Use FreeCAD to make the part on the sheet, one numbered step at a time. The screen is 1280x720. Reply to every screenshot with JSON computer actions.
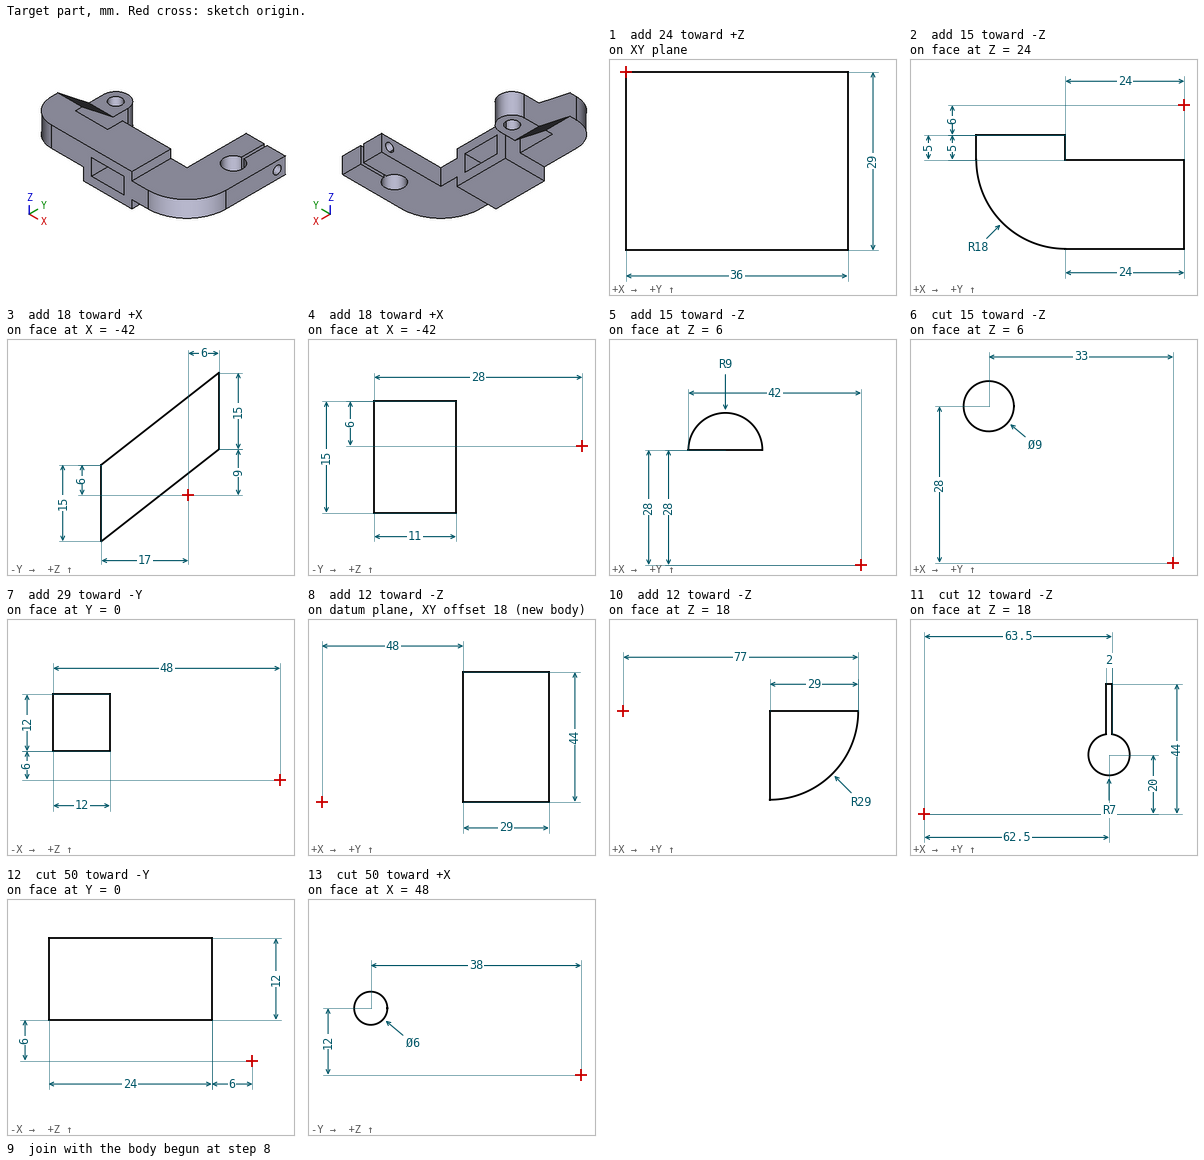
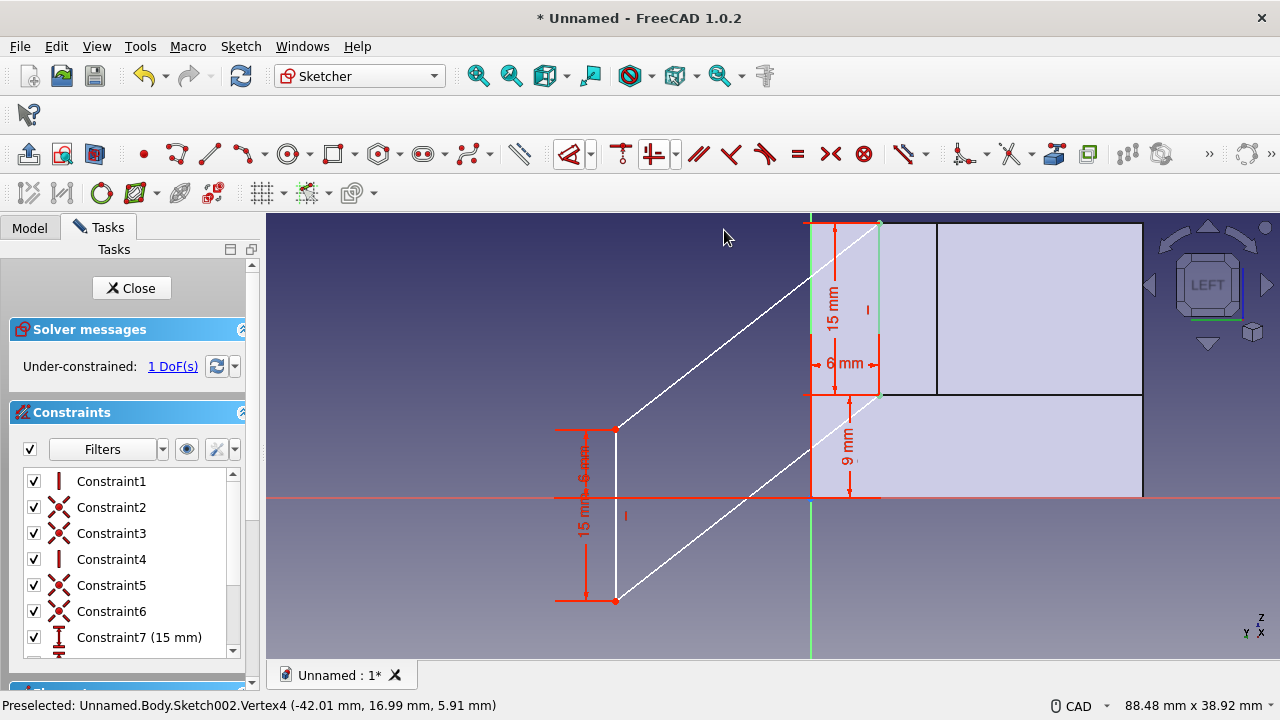
{"action": "left_click", "coordinate": [616, 430]}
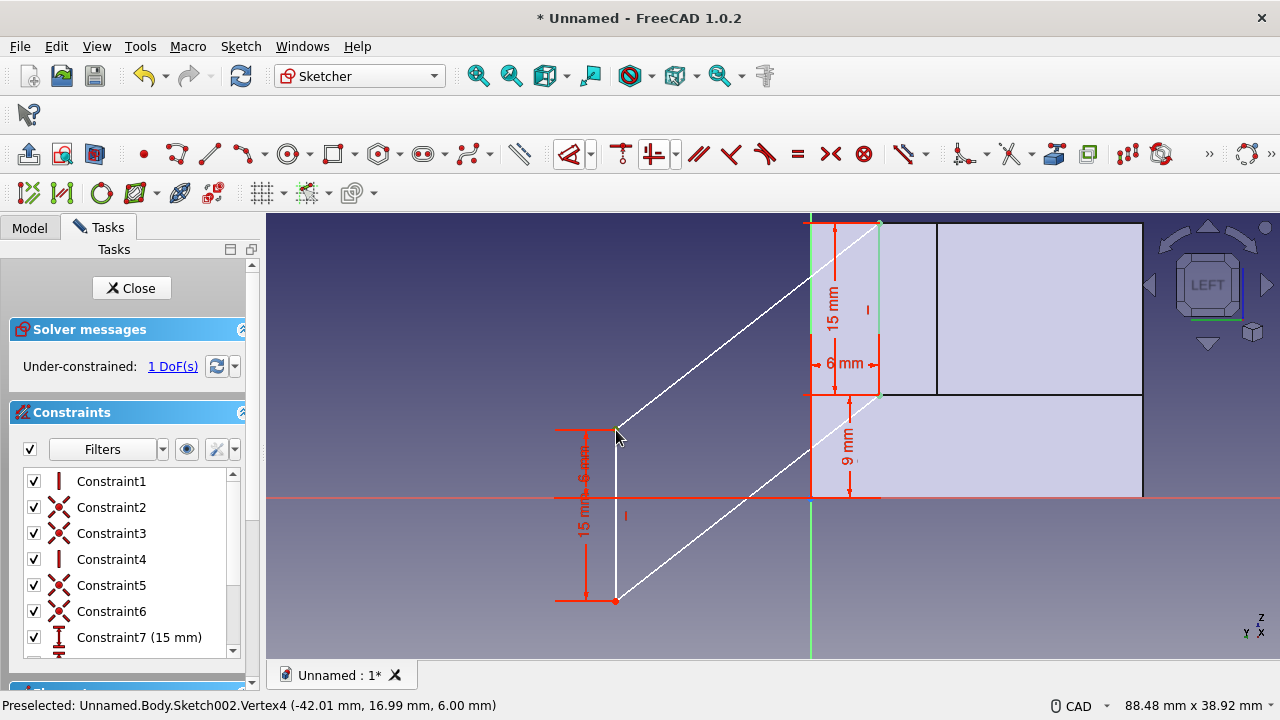
{"action": "left_click", "coordinate": [590, 154]}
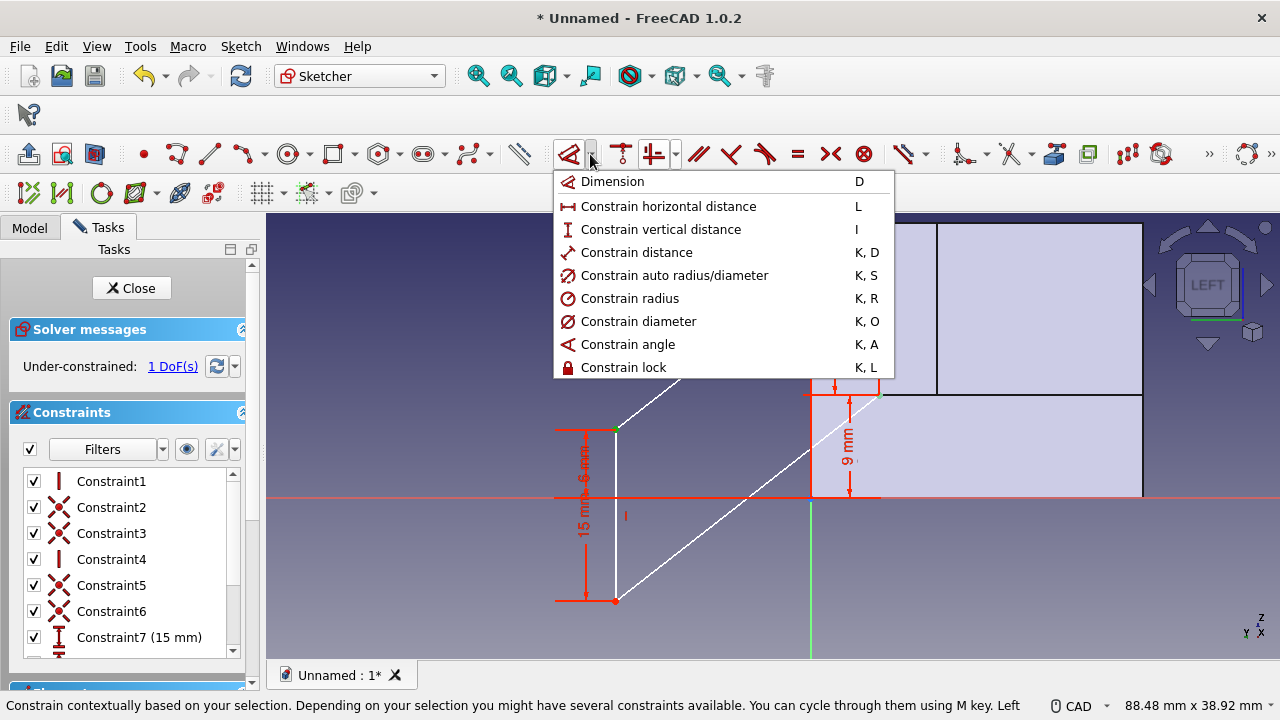
{"action": "left_click", "coordinate": [724, 206]}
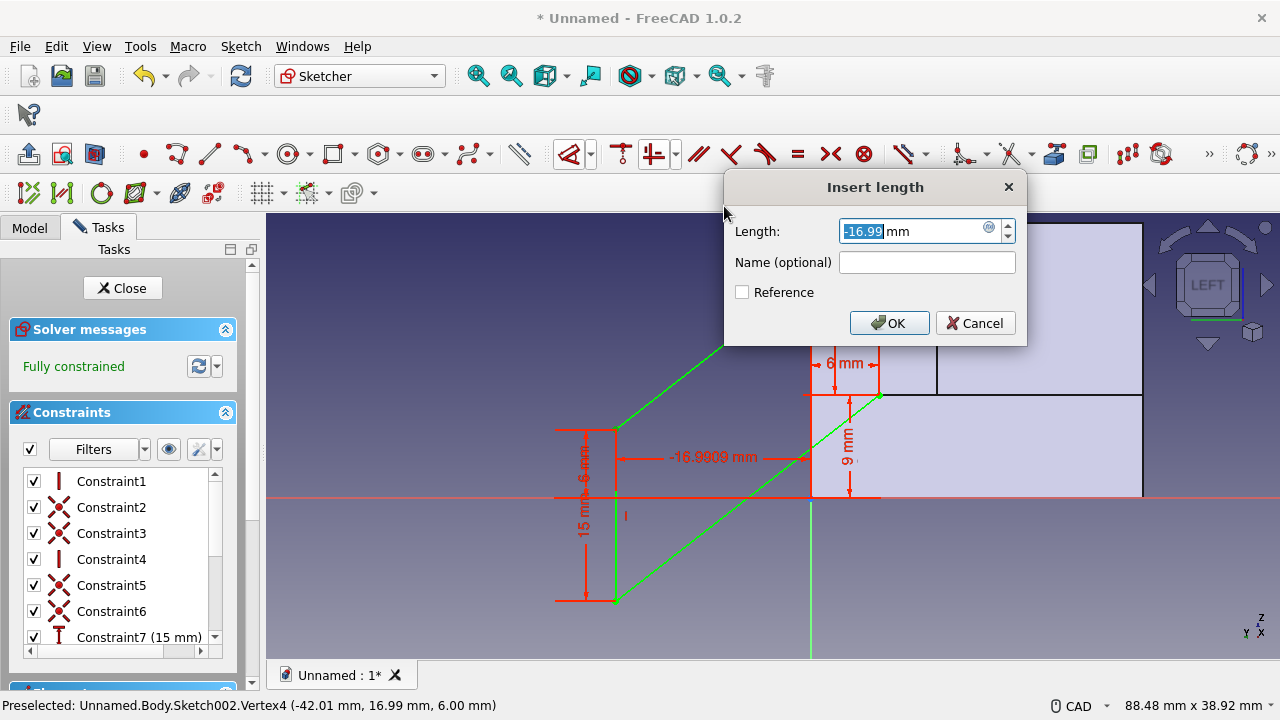
{"action": "type", "text": "-17"}
{"action": "key", "text": "Return"}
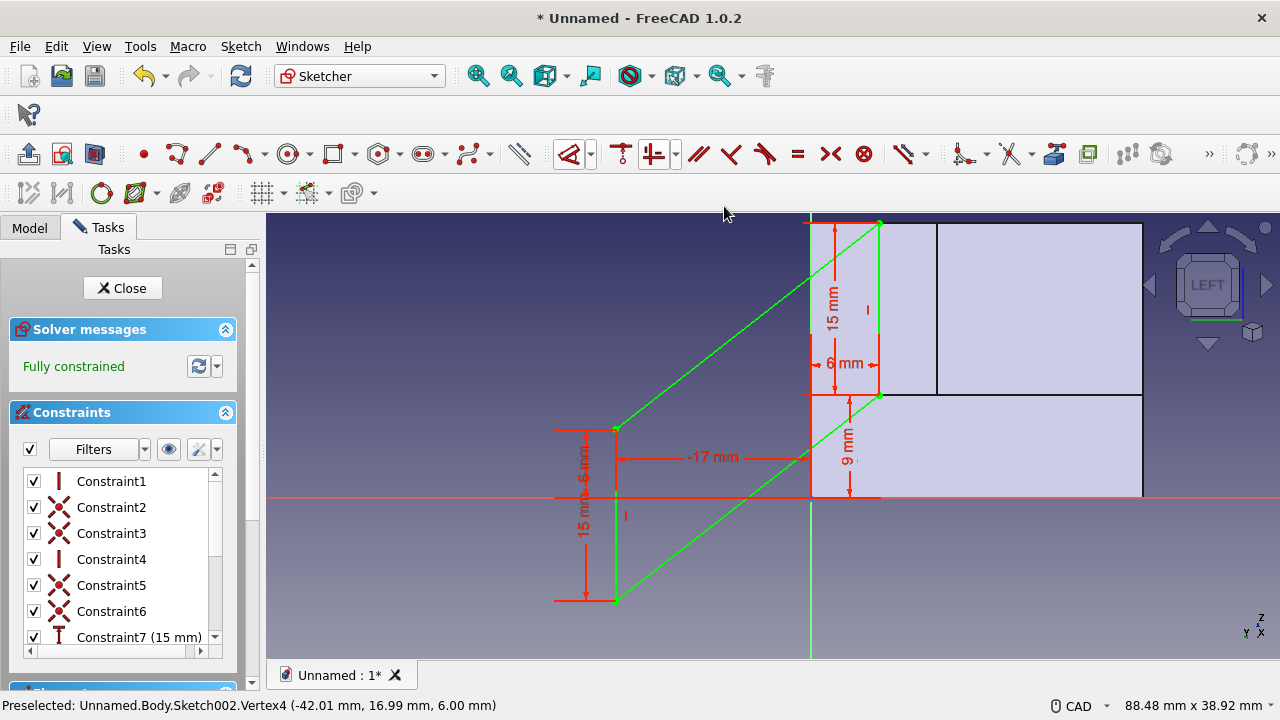
{"action": "left_click", "coordinate": [123, 288]}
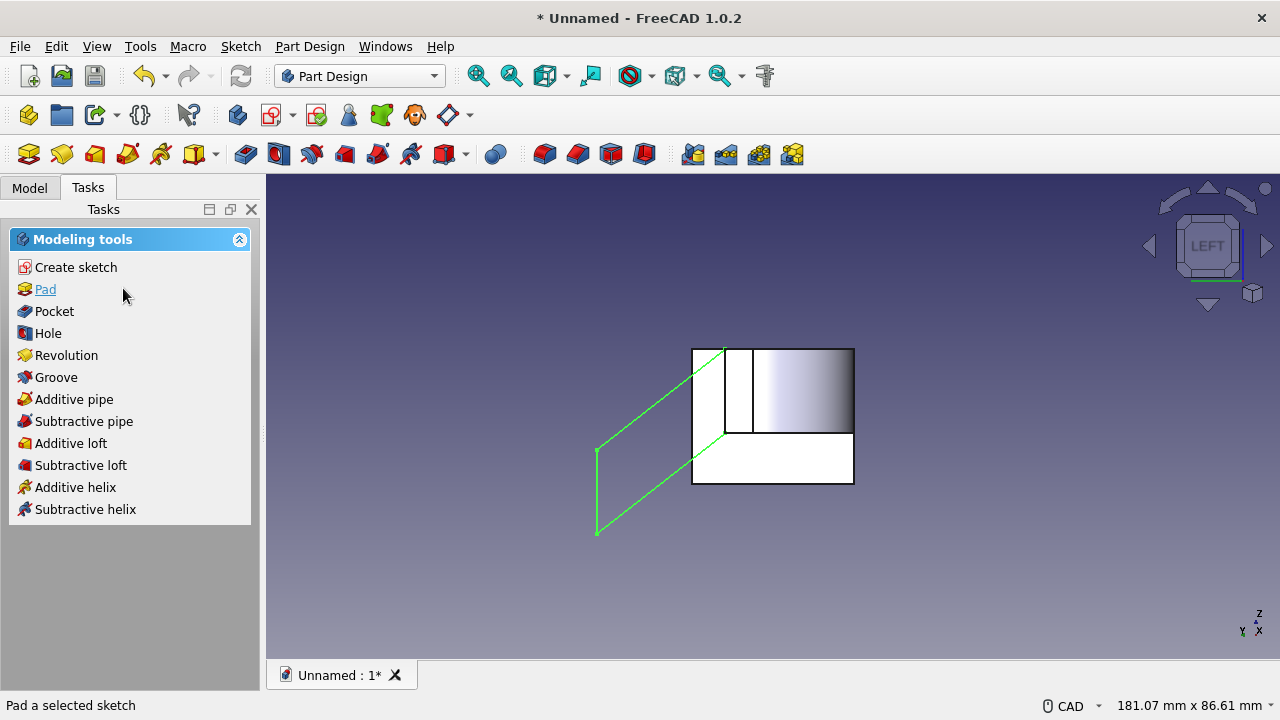
{"action": "left_click", "coordinate": [29, 154]}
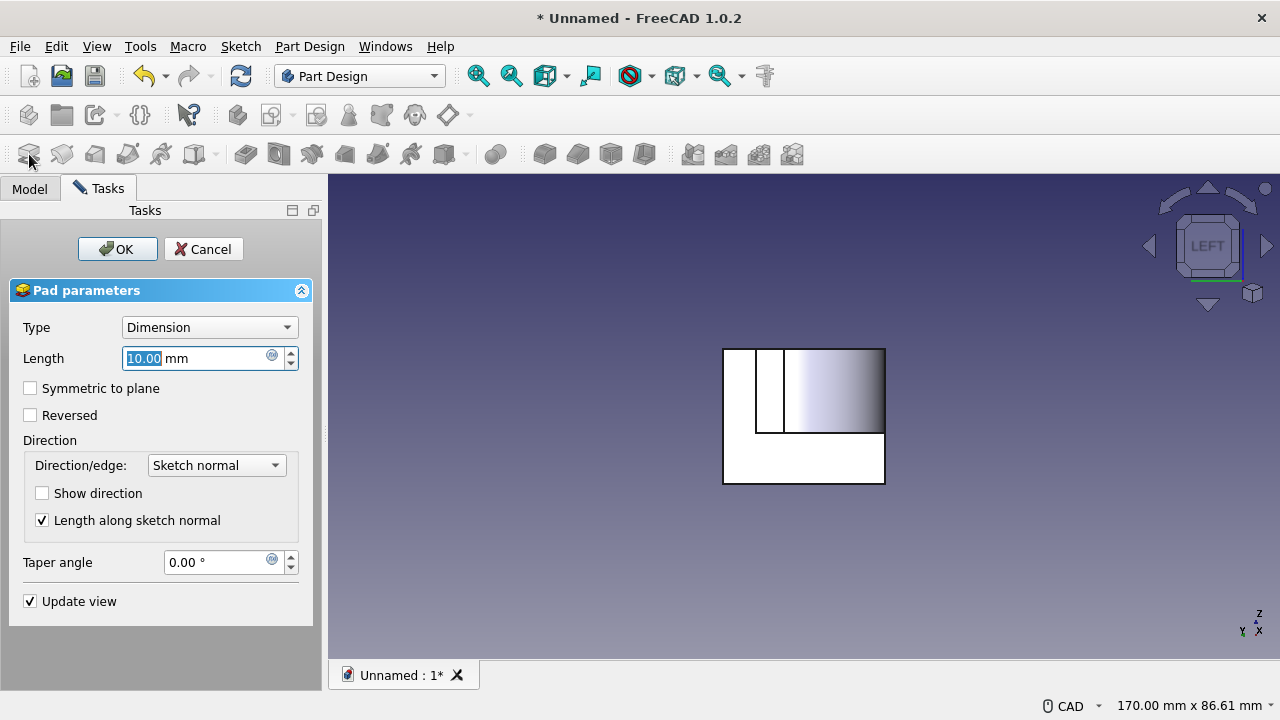
{"action": "type", "text": "18"}
{"action": "key", "text": "Tab"}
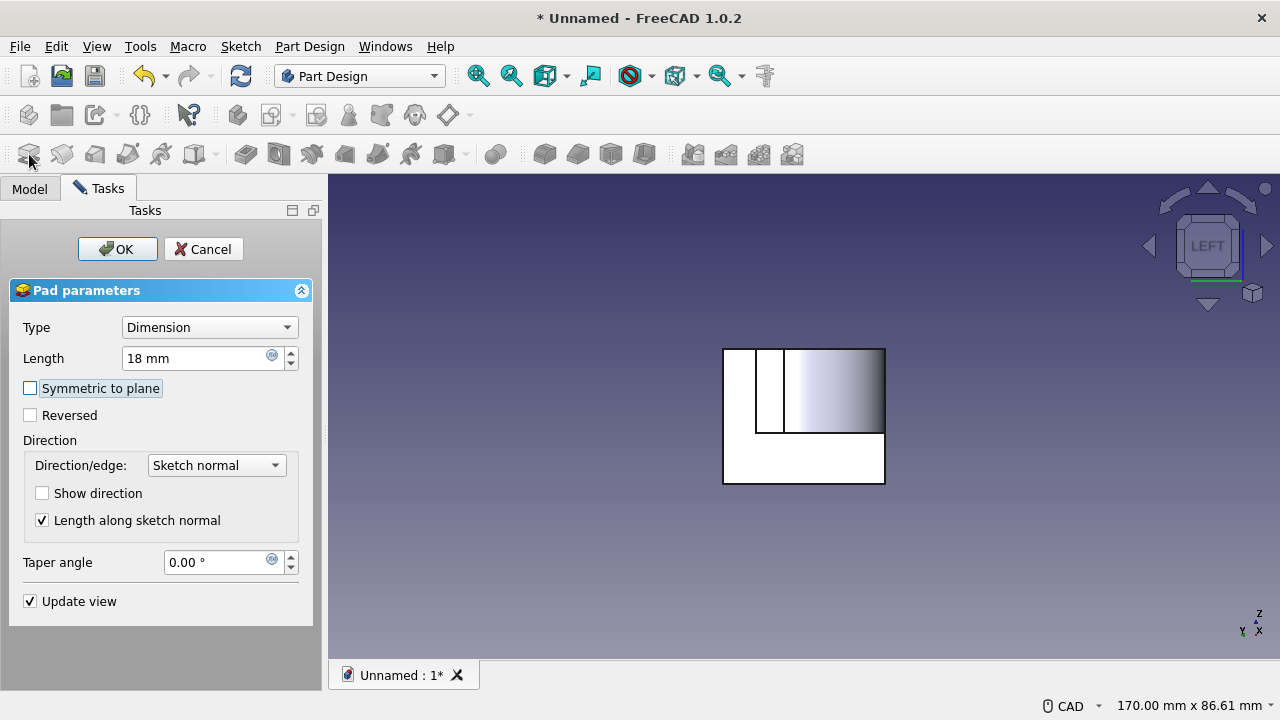
{"action": "left_click", "coordinate": [31, 415]}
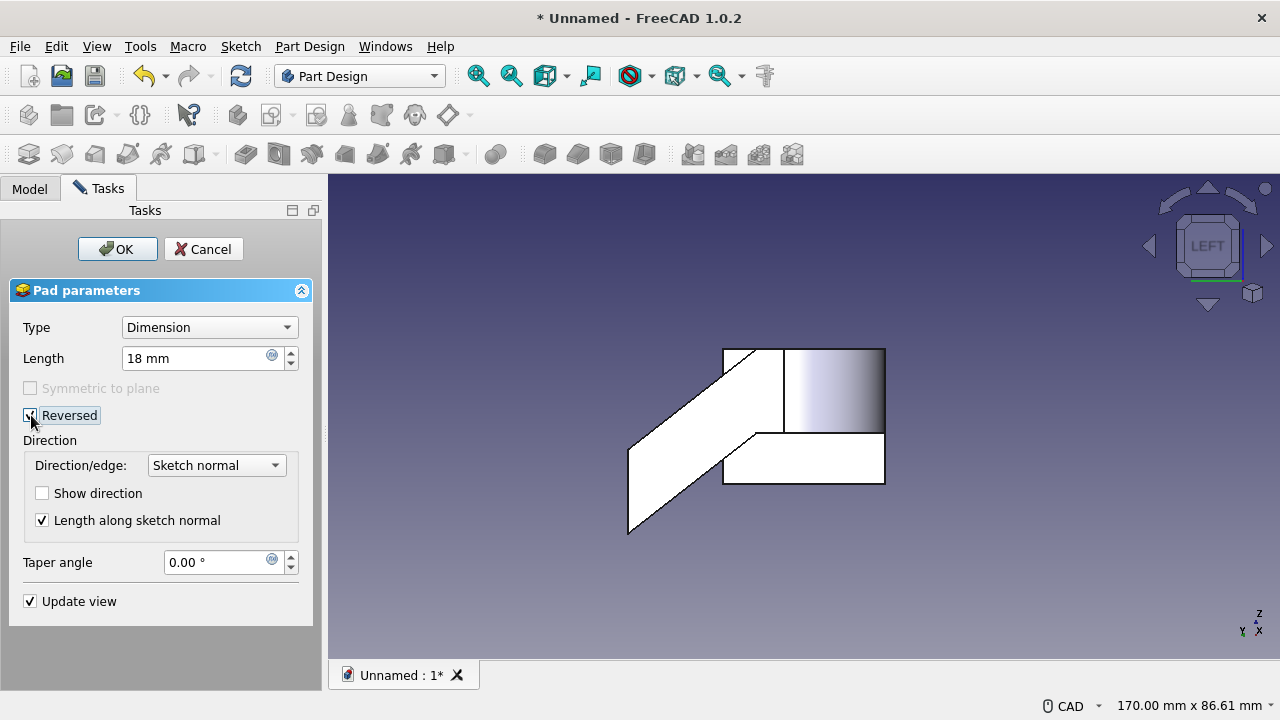
{"action": "left_click", "coordinate": [118, 249]}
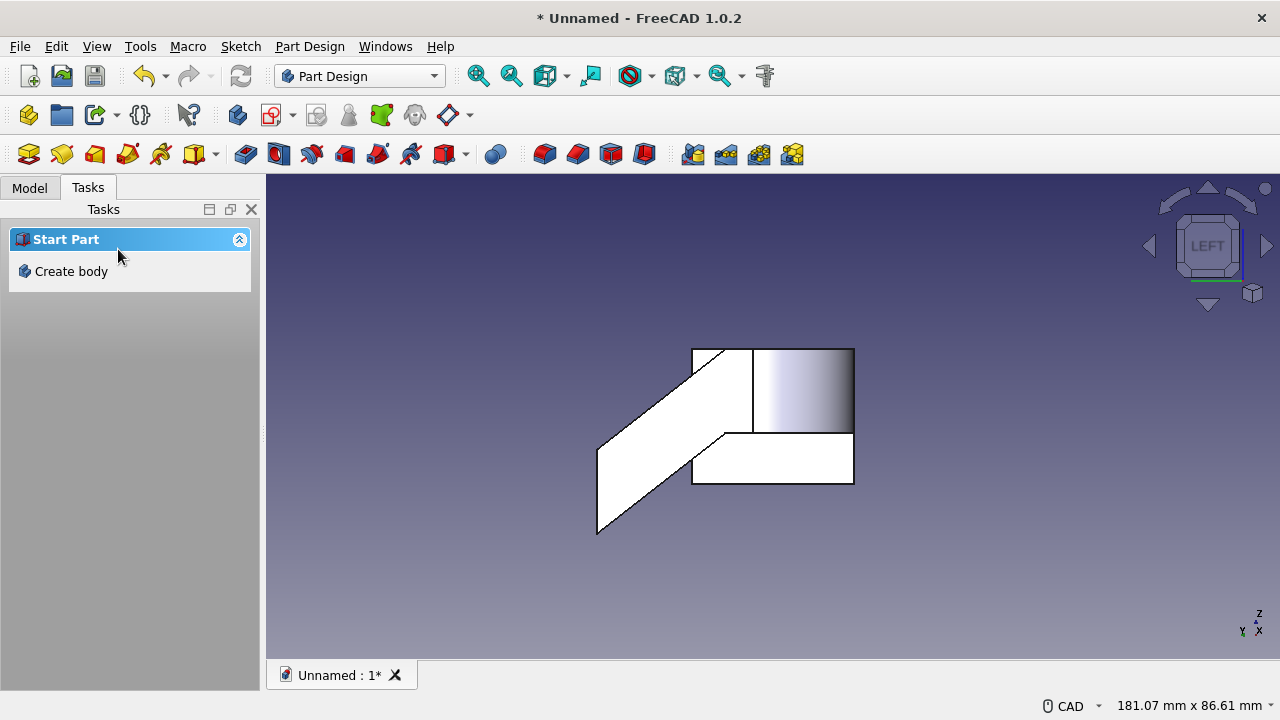
{"action": "left_click", "coordinate": [479, 76]}